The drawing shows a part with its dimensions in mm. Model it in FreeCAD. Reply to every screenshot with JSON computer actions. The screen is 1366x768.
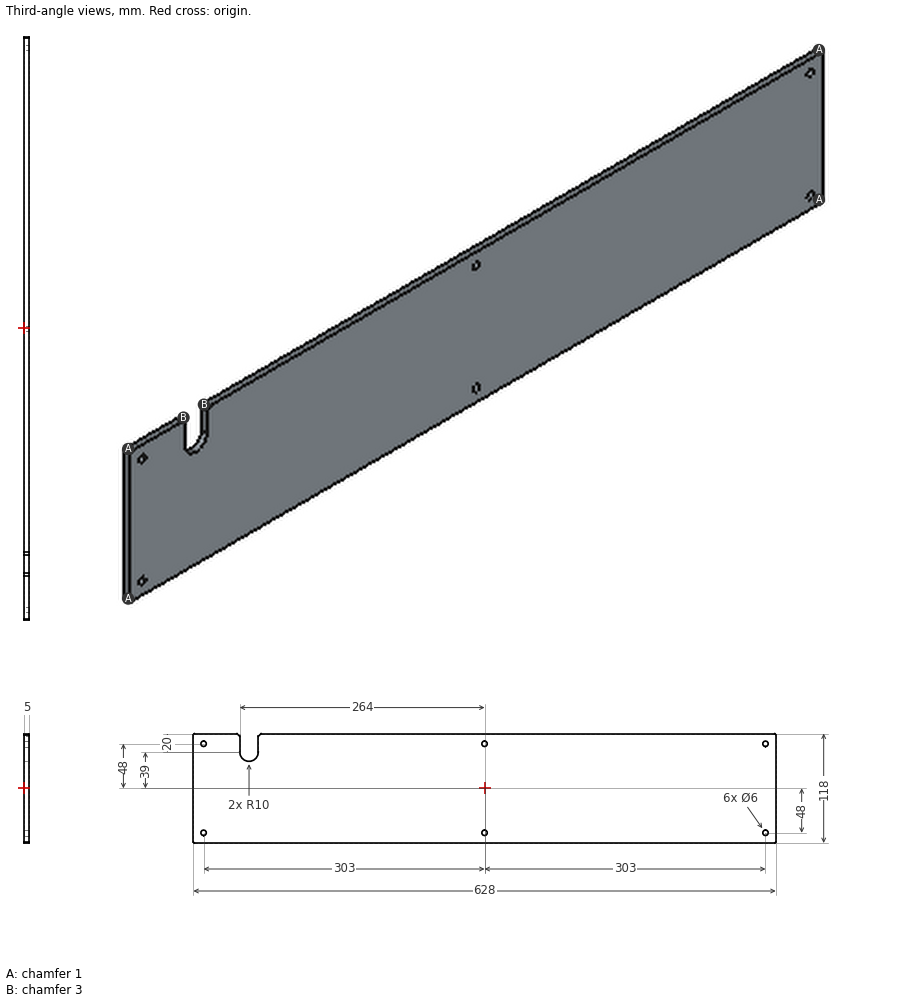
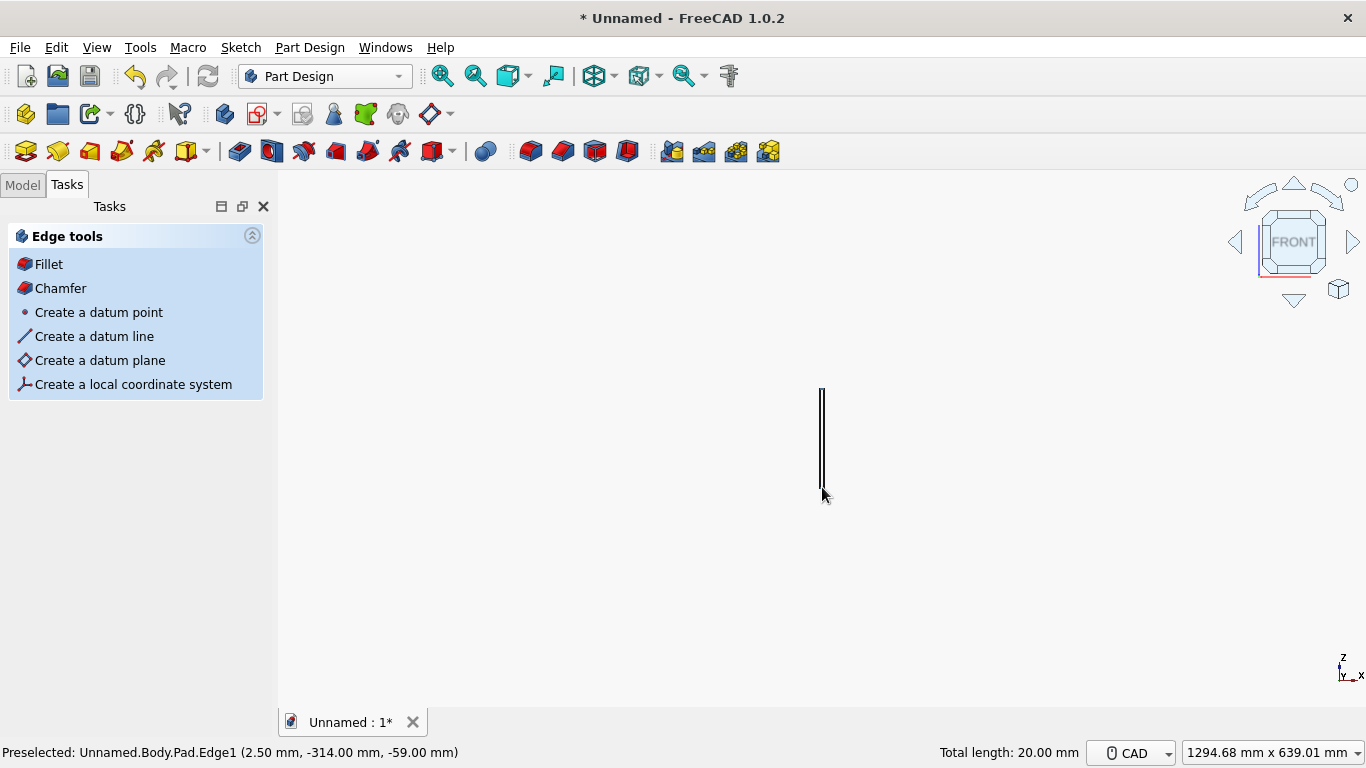
{"action": "key", "text": "v 1"}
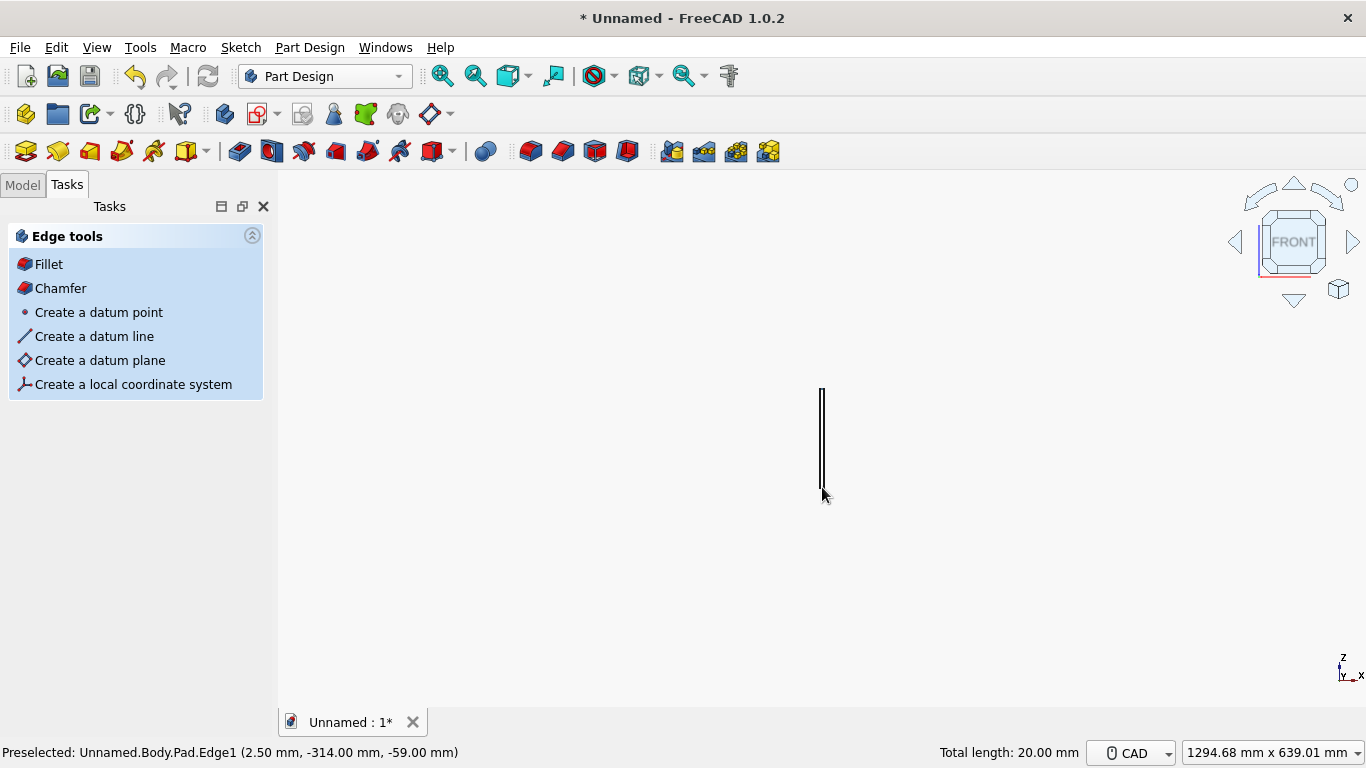
{"action": "left_click", "coordinate": [564, 152]}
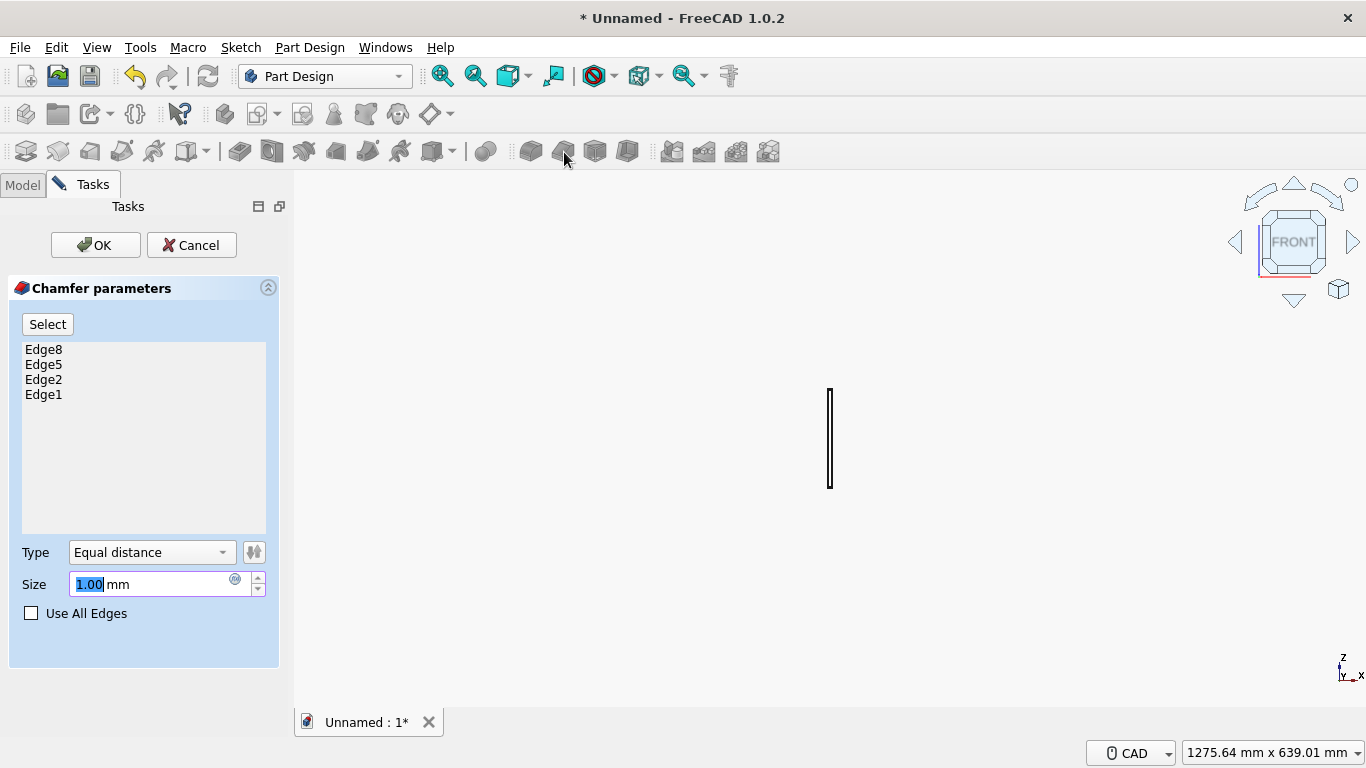
{"action": "type", "text": "1"}
{"action": "key", "text": "Tab"}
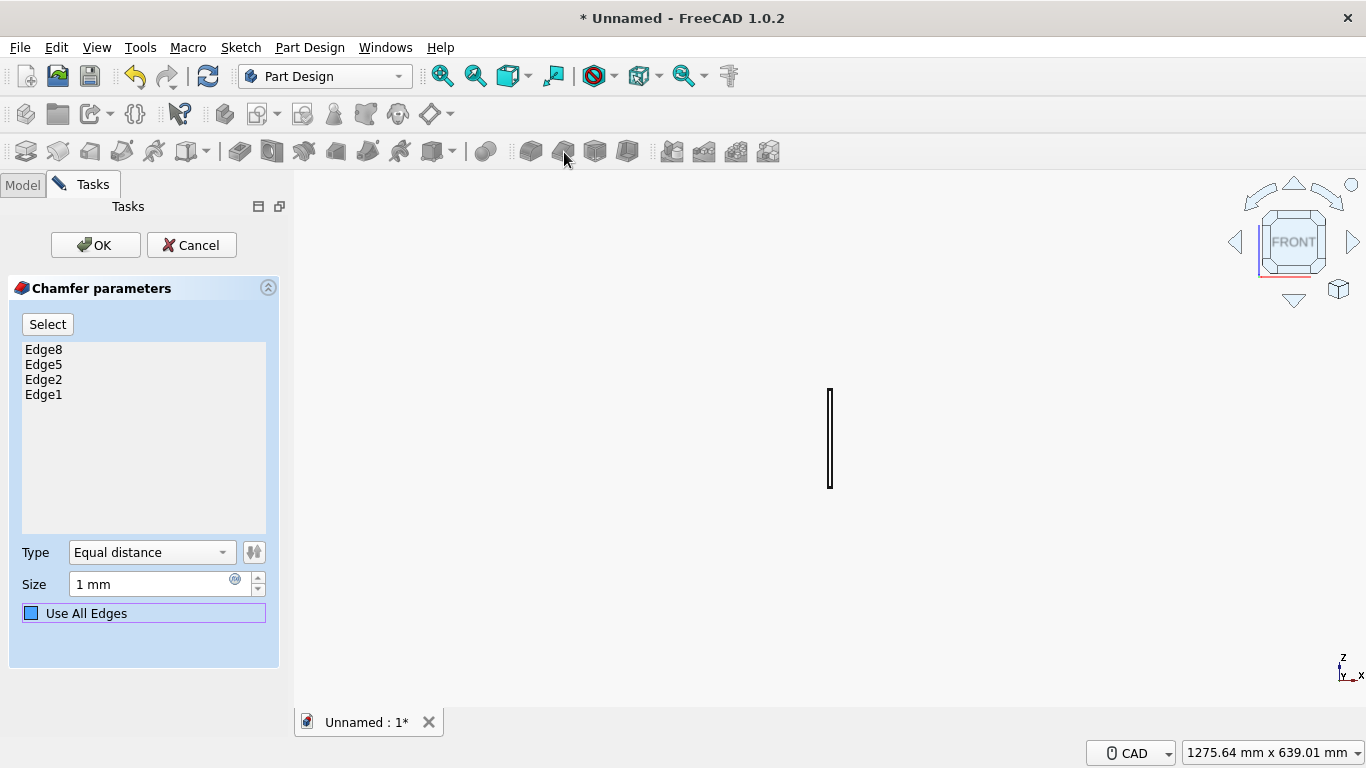
{"action": "left_click", "coordinate": [96, 245]}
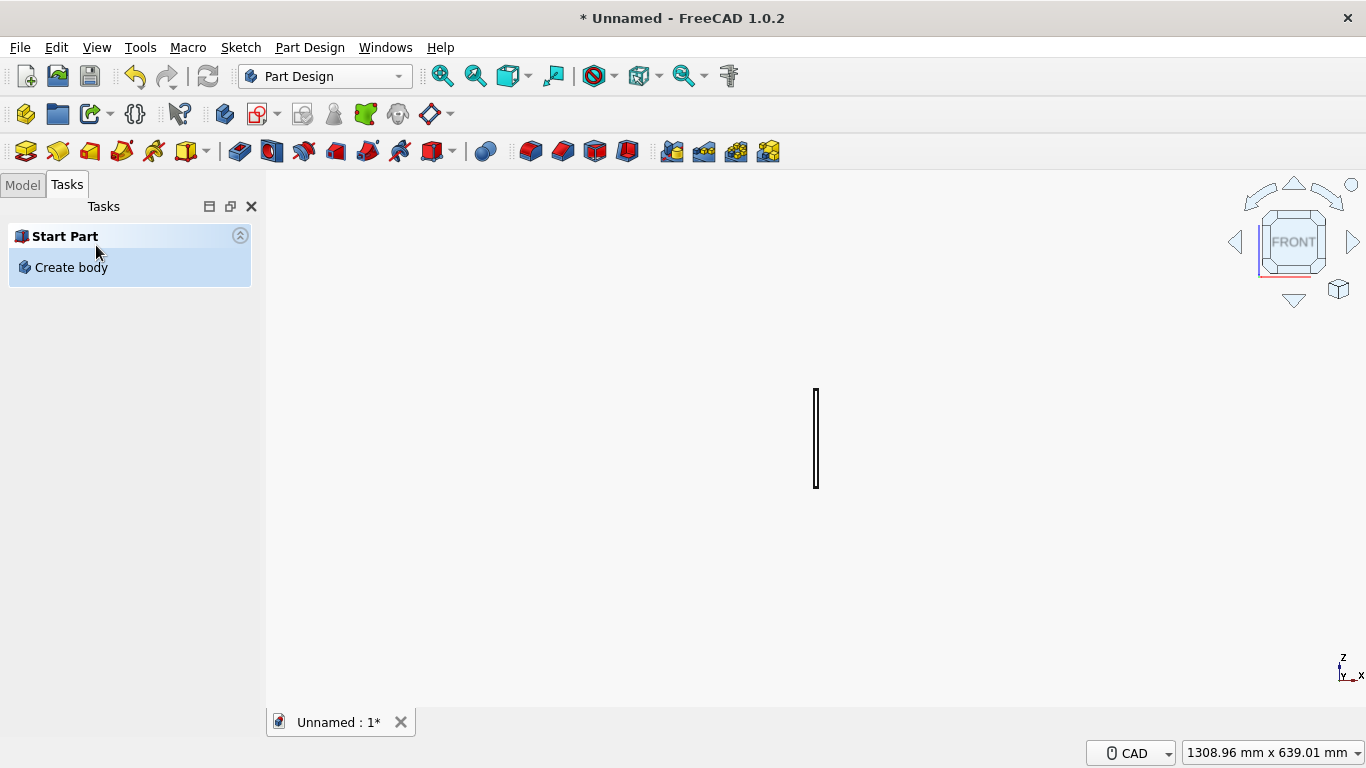
{"action": "left_click", "coordinate": [444, 76]}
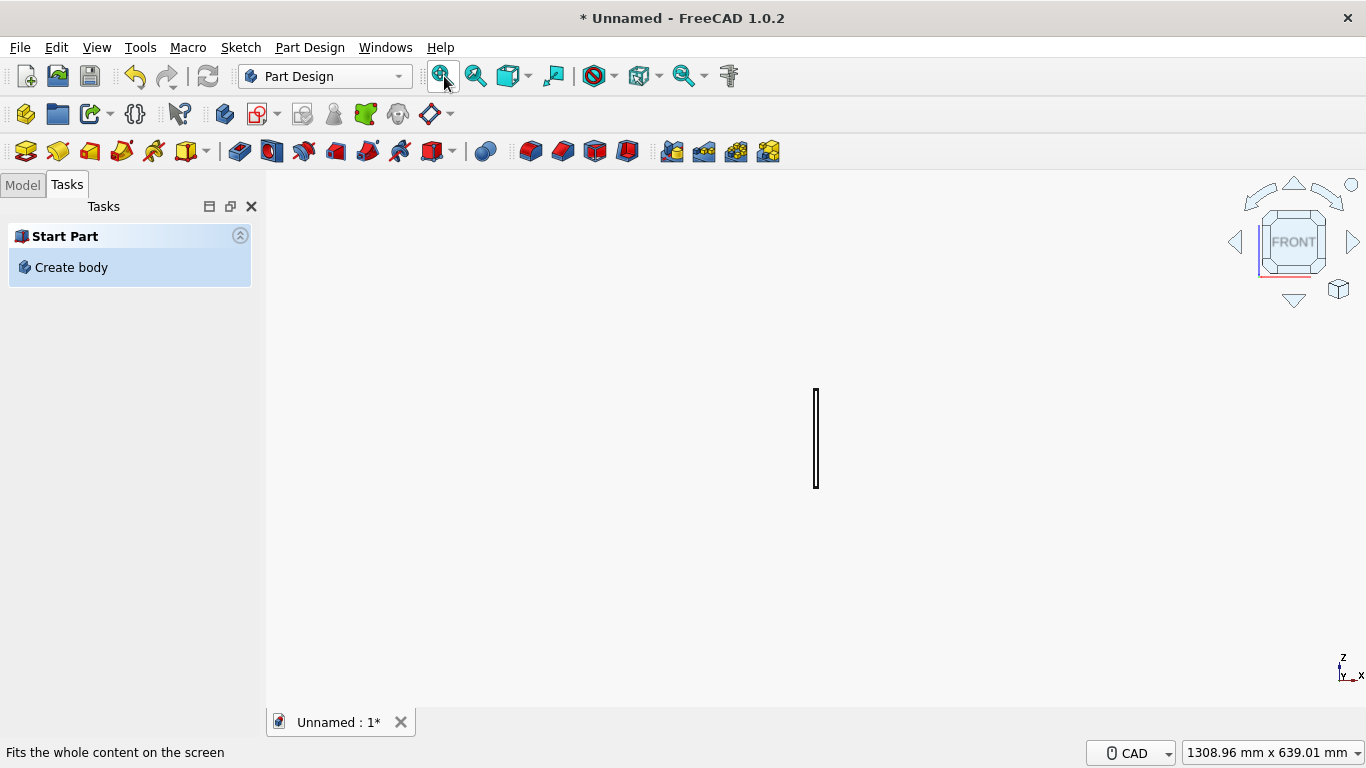
{"action": "left_click", "coordinate": [258, 114]}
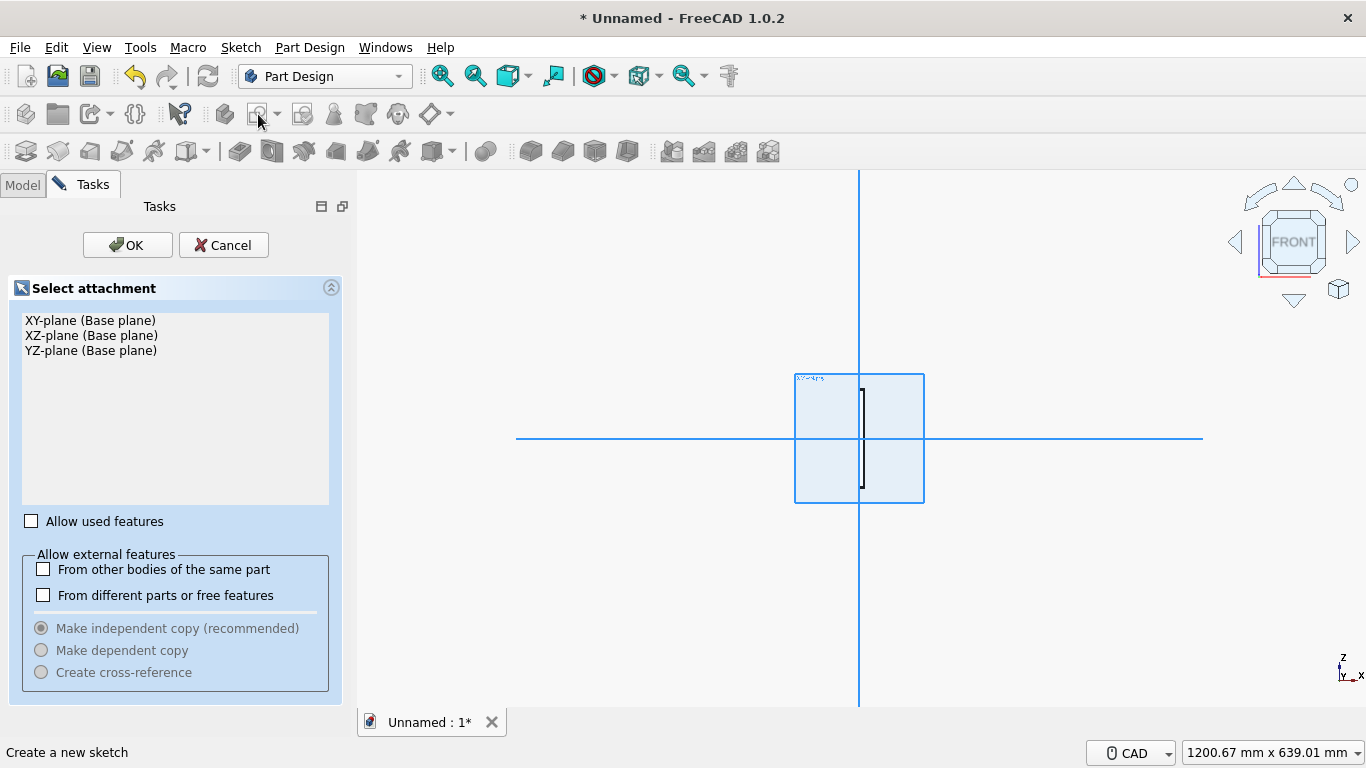
{"action": "left_click", "coordinate": [82, 350]}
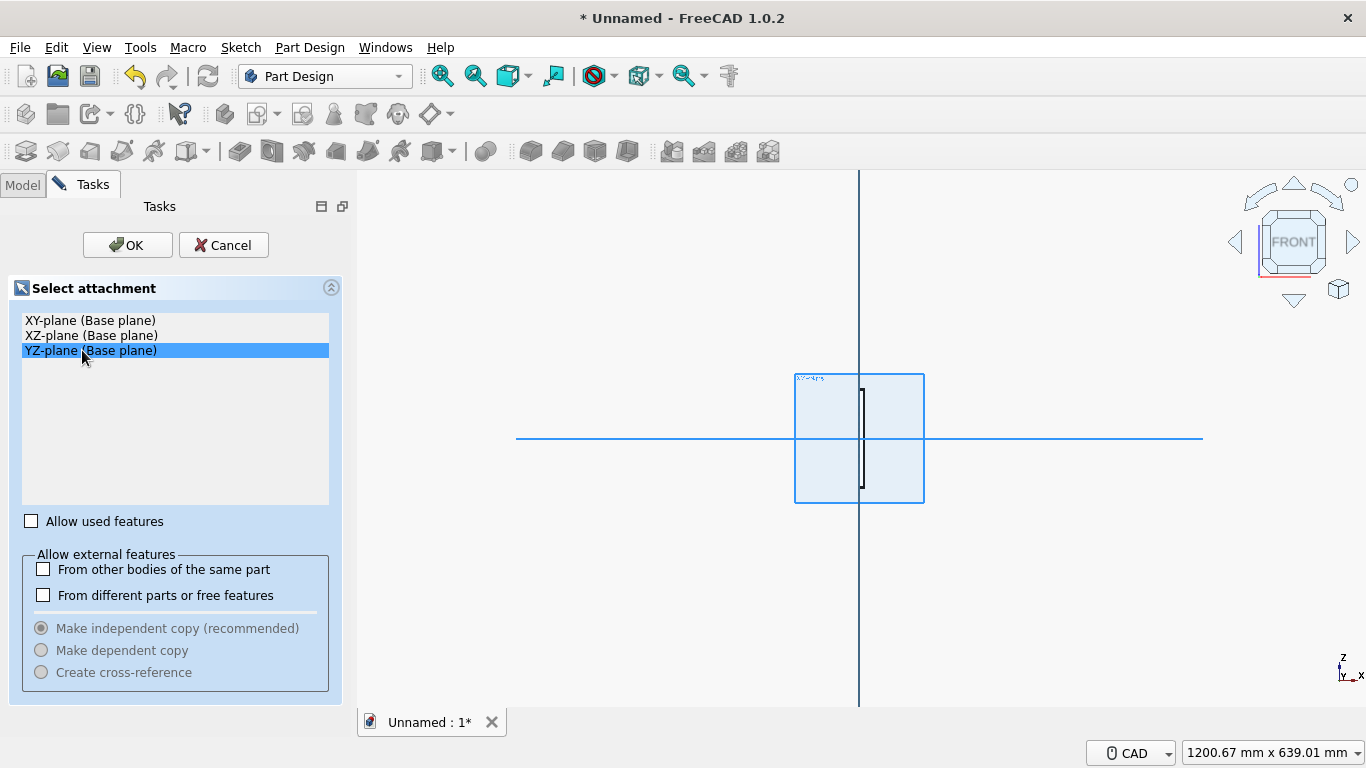
{"action": "left_click", "coordinate": [128, 245]}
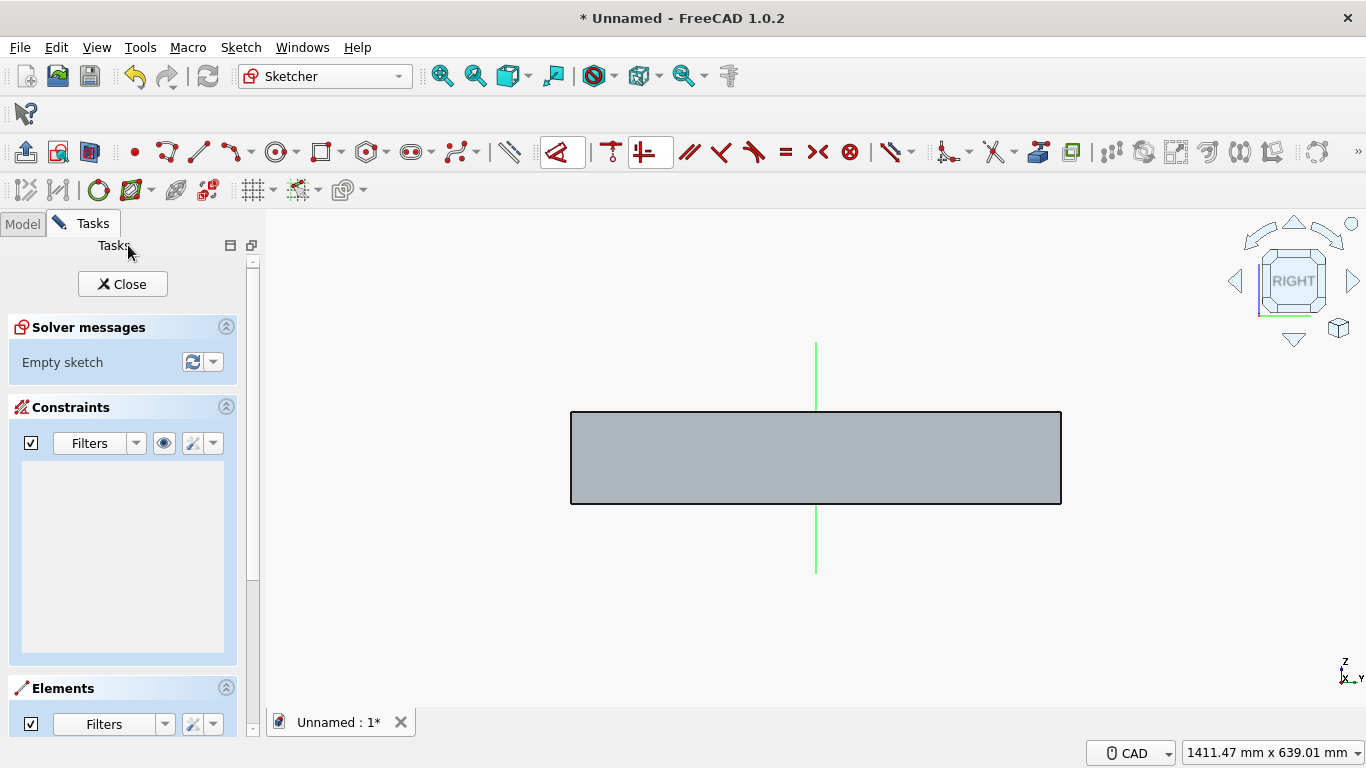
{"action": "left_click", "coordinate": [90, 152]}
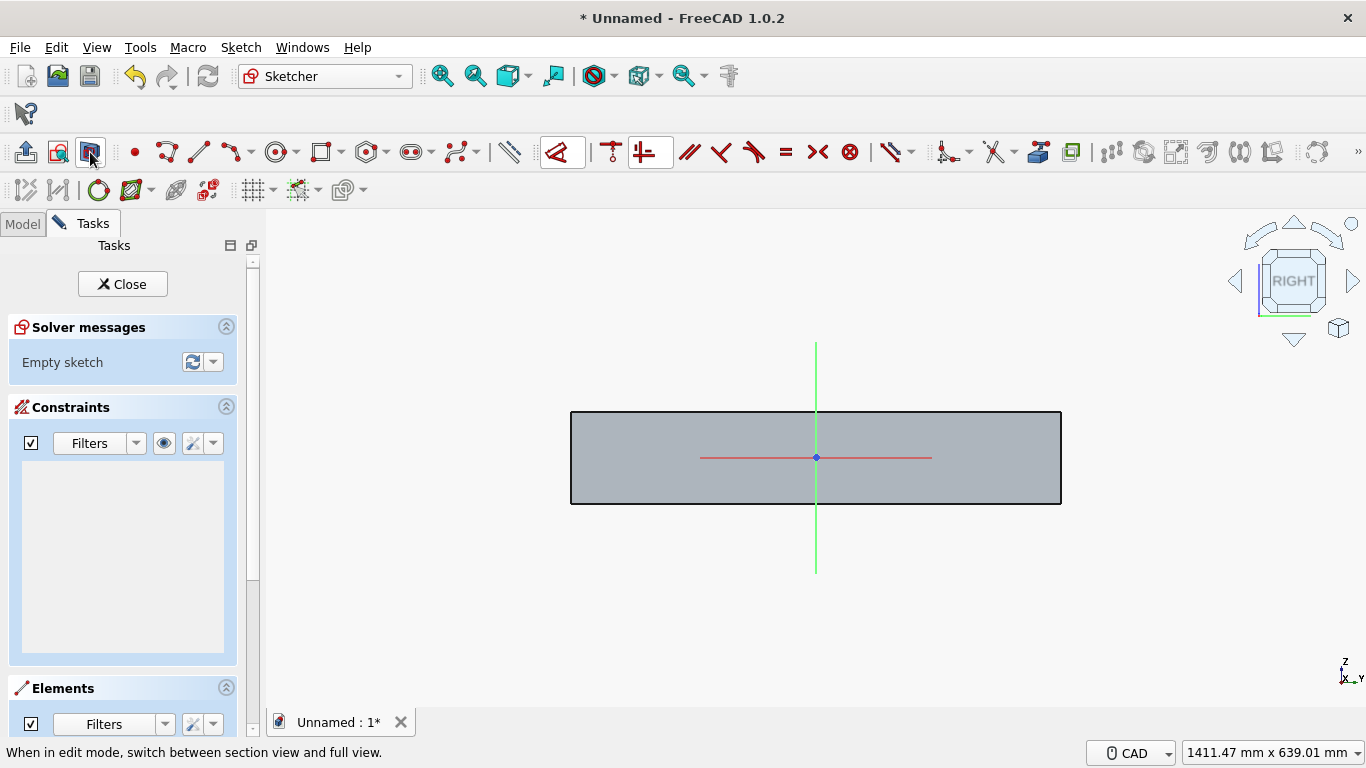
{"action": "key", "text": "g c"}